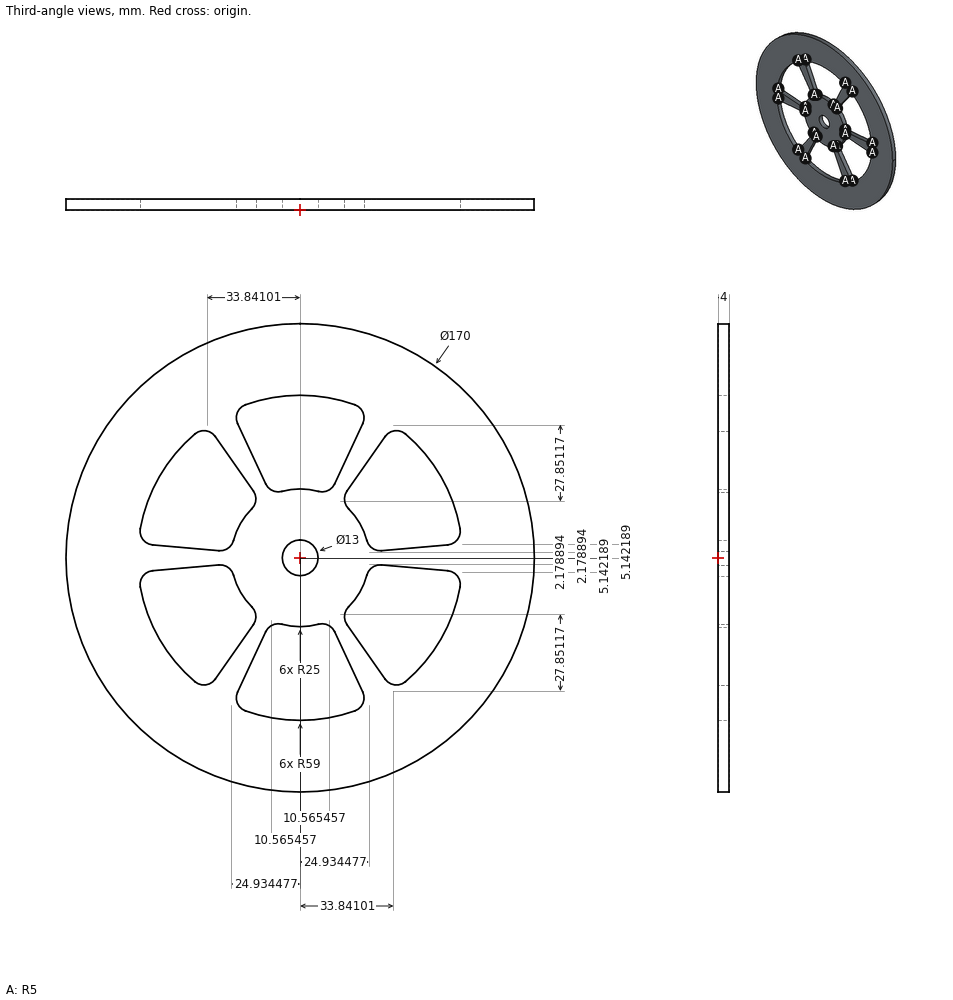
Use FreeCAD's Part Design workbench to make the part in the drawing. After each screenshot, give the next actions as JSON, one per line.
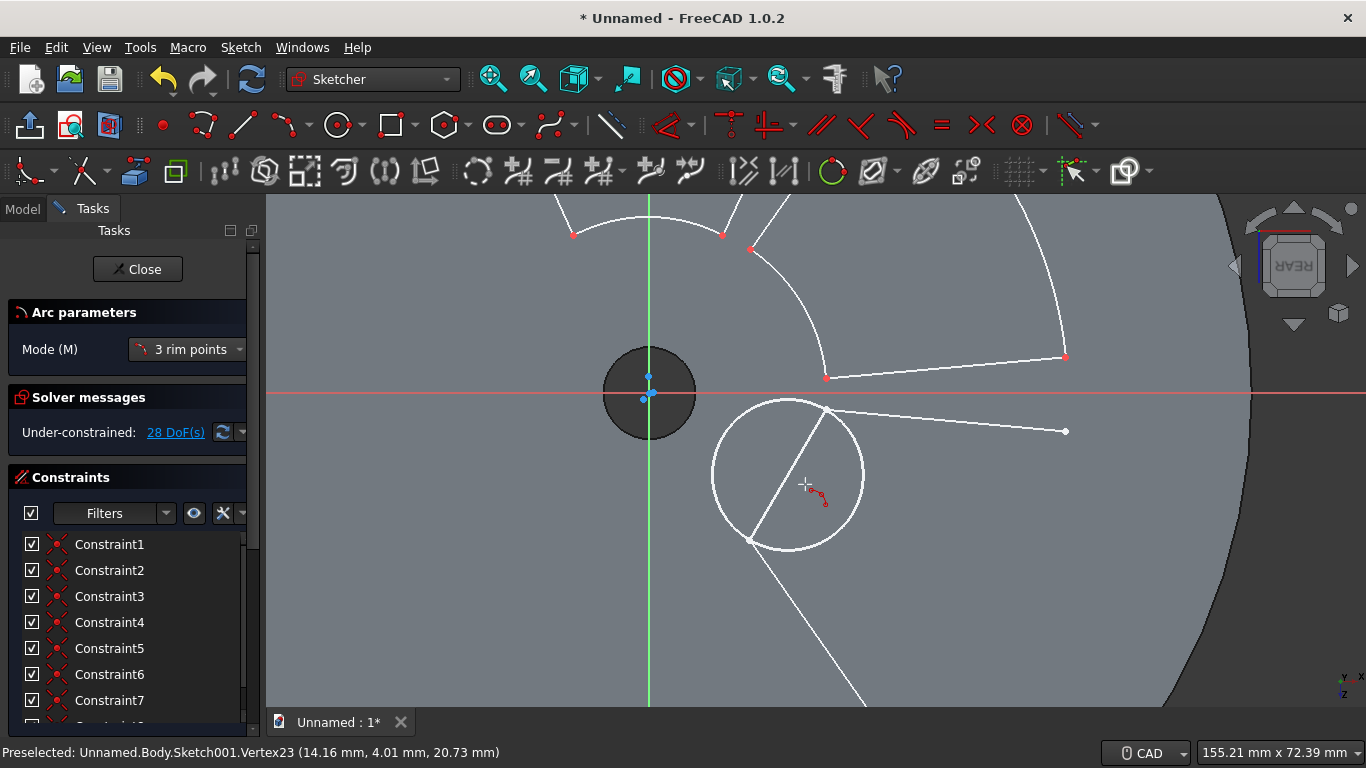
{"action": "left_click", "coordinate": [803, 482]}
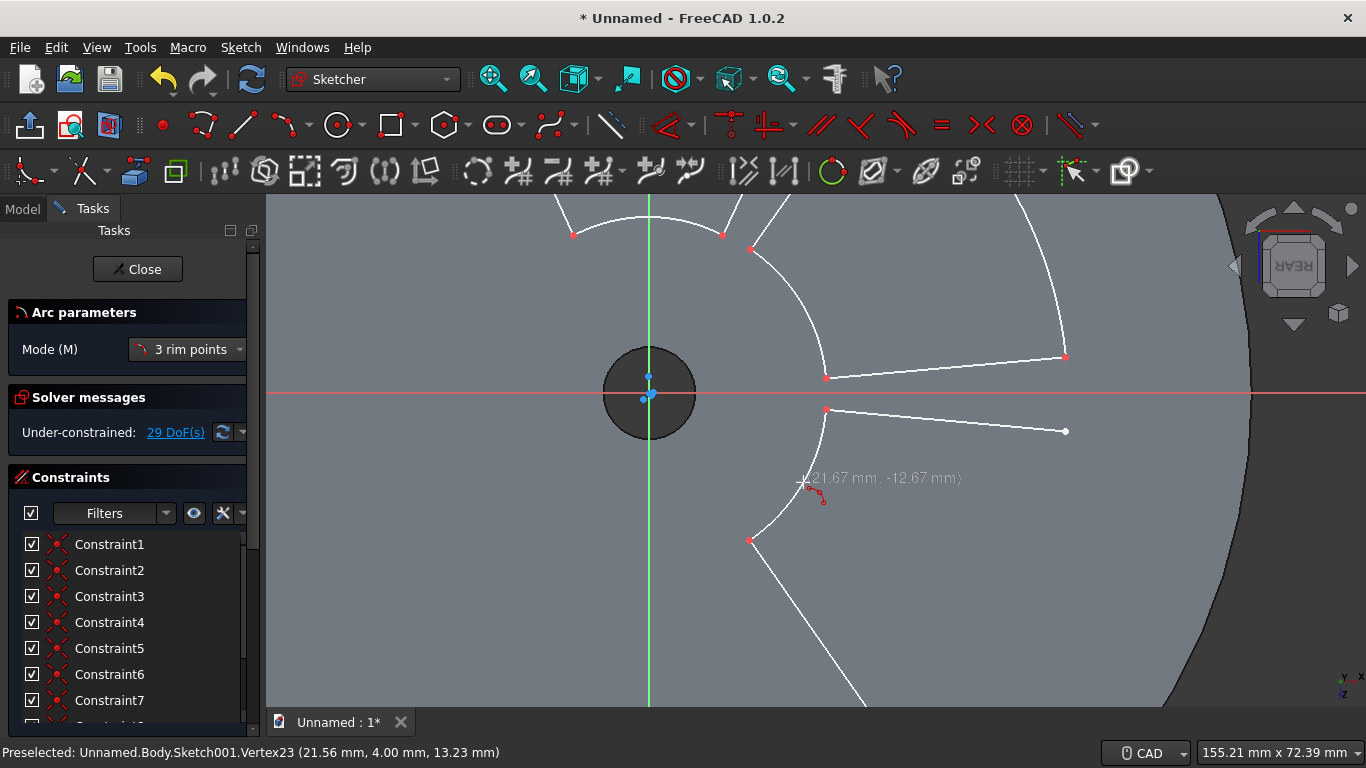
{"action": "scroll", "coordinate": [805, 484], "scroll_direction": "down", "scroll_amount": 5}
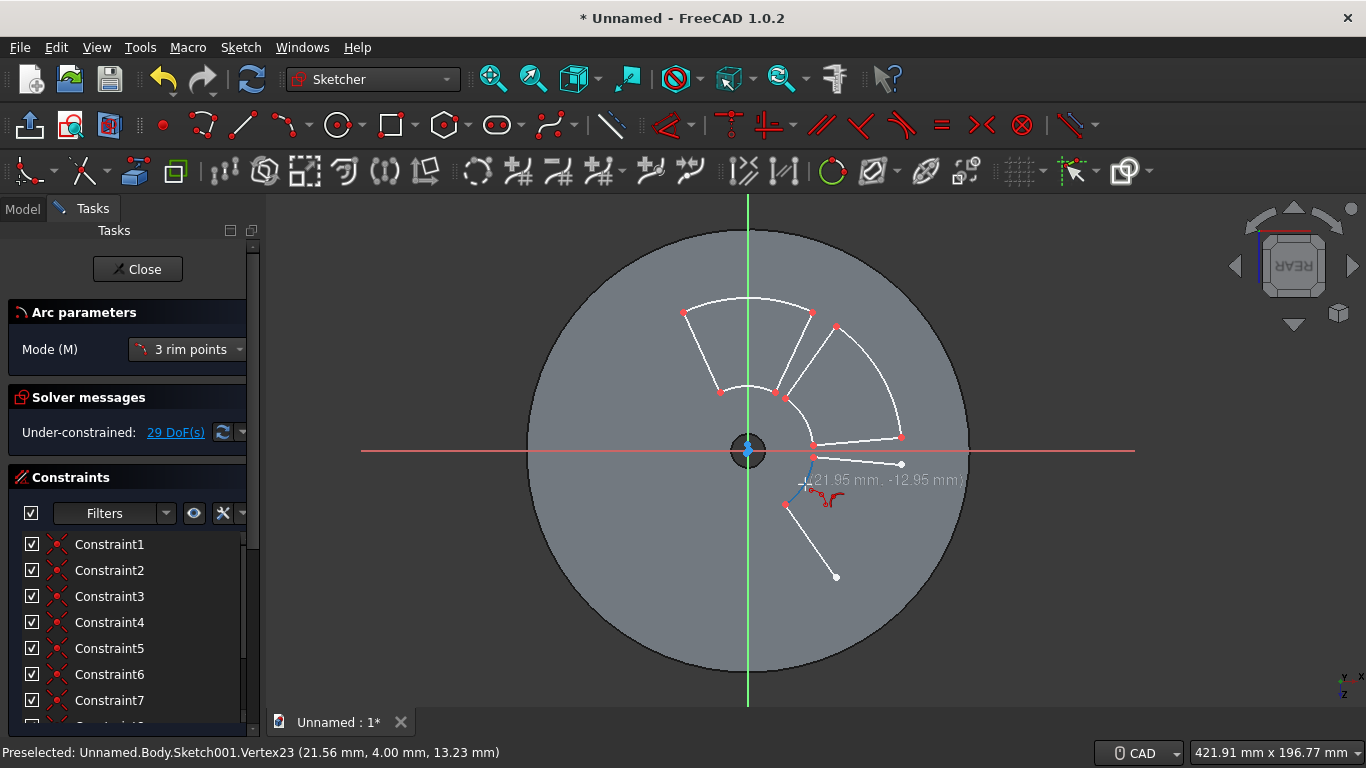
{"action": "left_click", "coordinate": [836, 578]}
{"action": "left_click", "coordinate": [901, 465]}
{"action": "left_click", "coordinate": [881, 528]}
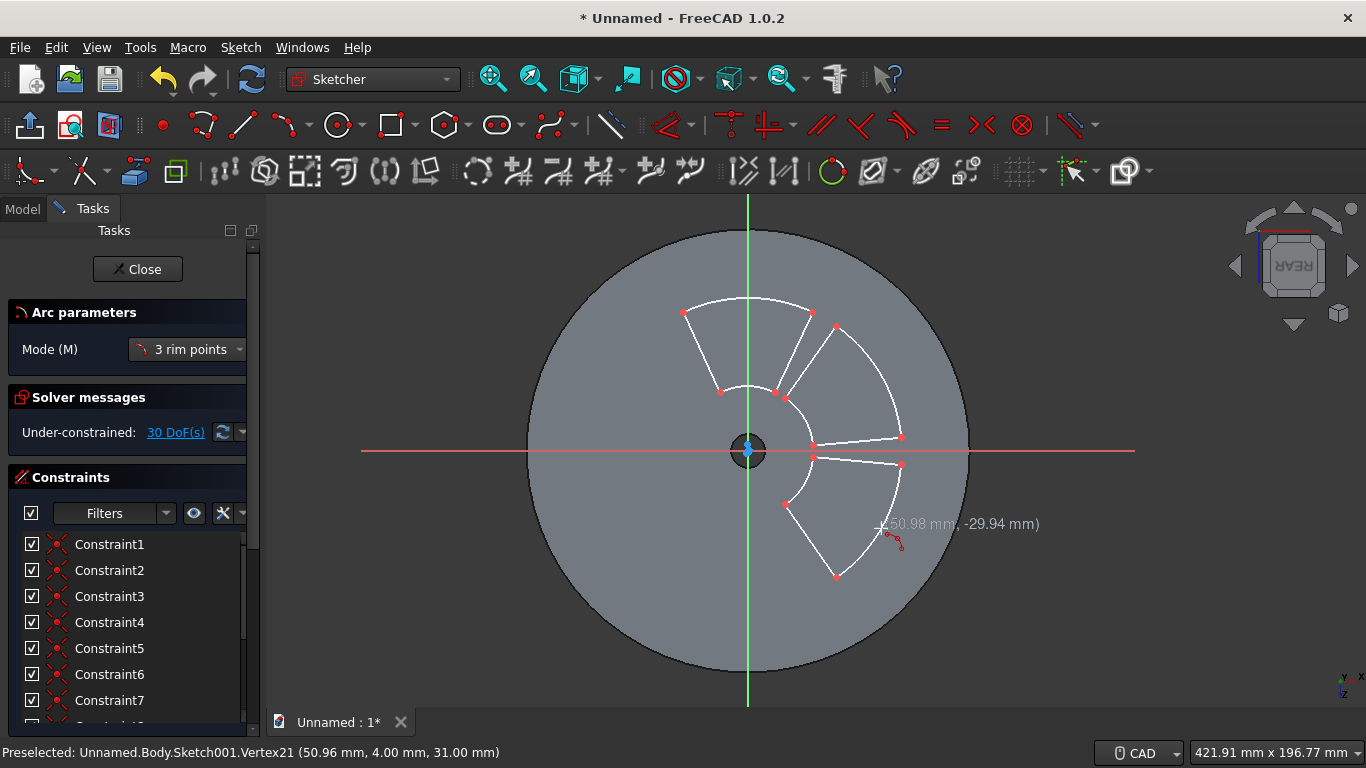
{"action": "left_click", "coordinate": [244, 126]}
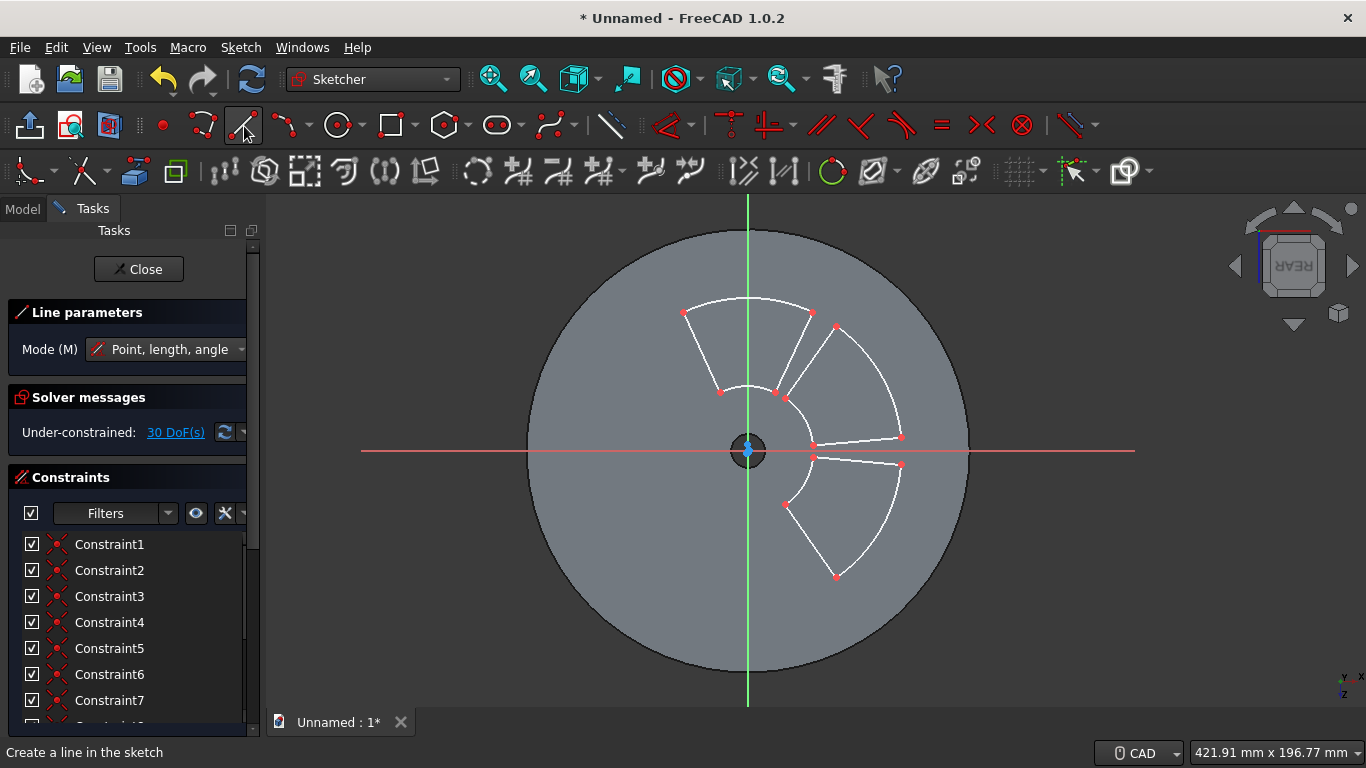
{"action": "left_click", "coordinate": [813, 590]}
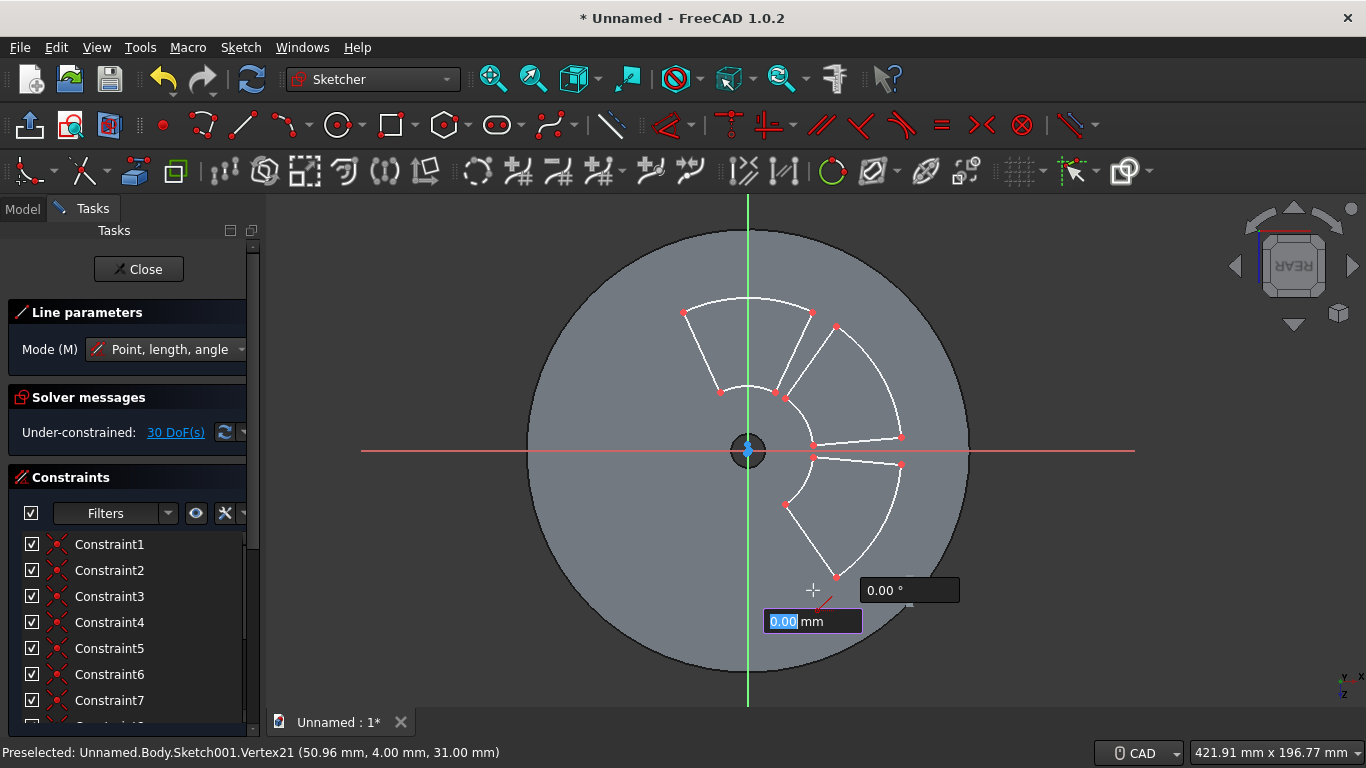
{"action": "scroll", "coordinate": [776, 510], "scroll_direction": "up", "scroll_amount": 2}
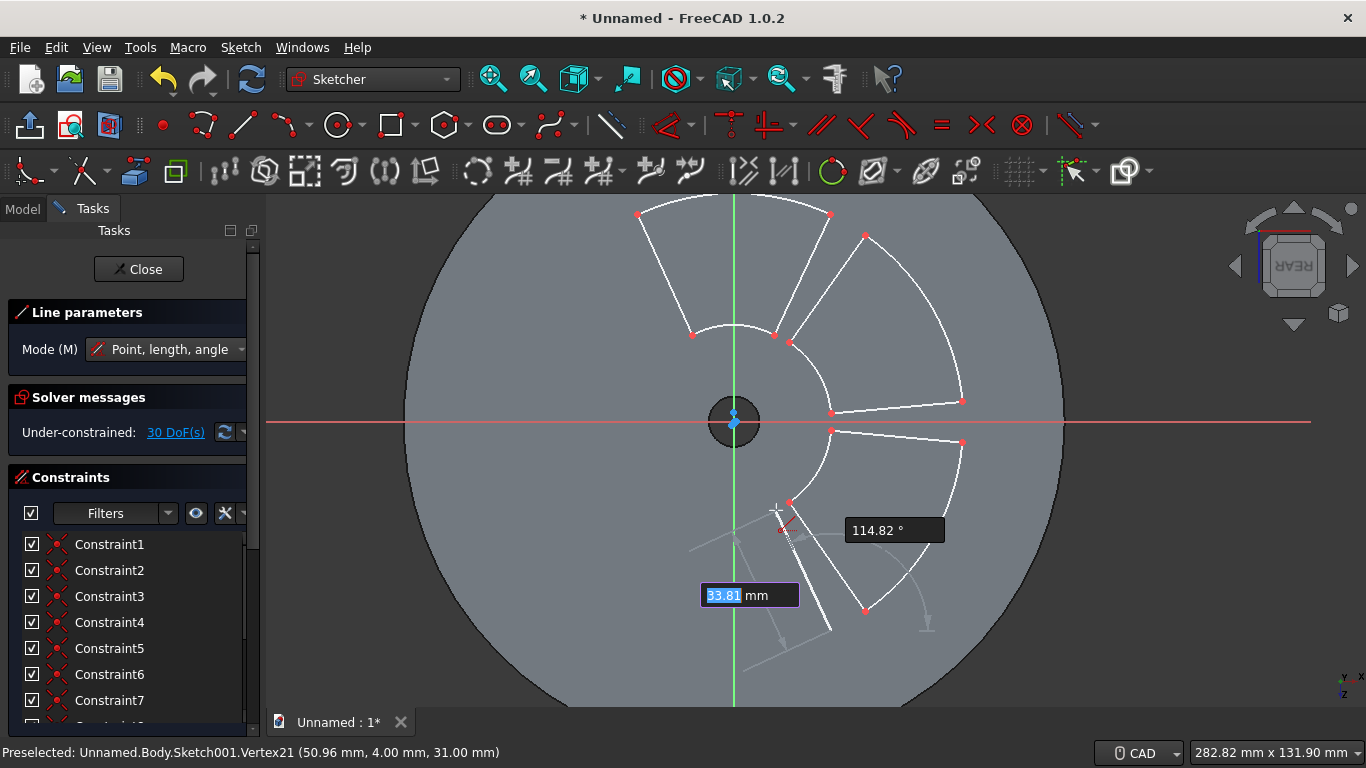
{"action": "left_click", "coordinate": [775, 510]}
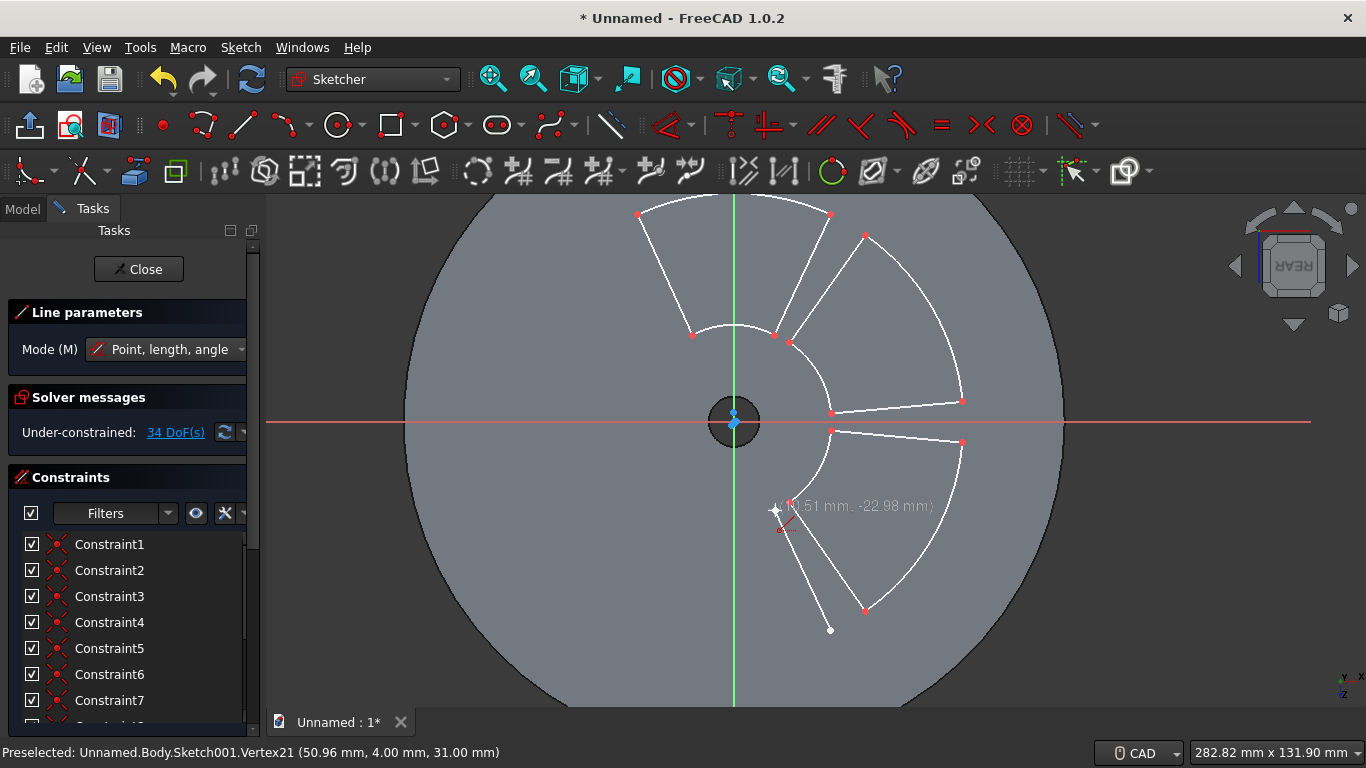
{"action": "left_click", "coordinate": [693, 510]}
{"action": "left_click", "coordinate": [637, 630]}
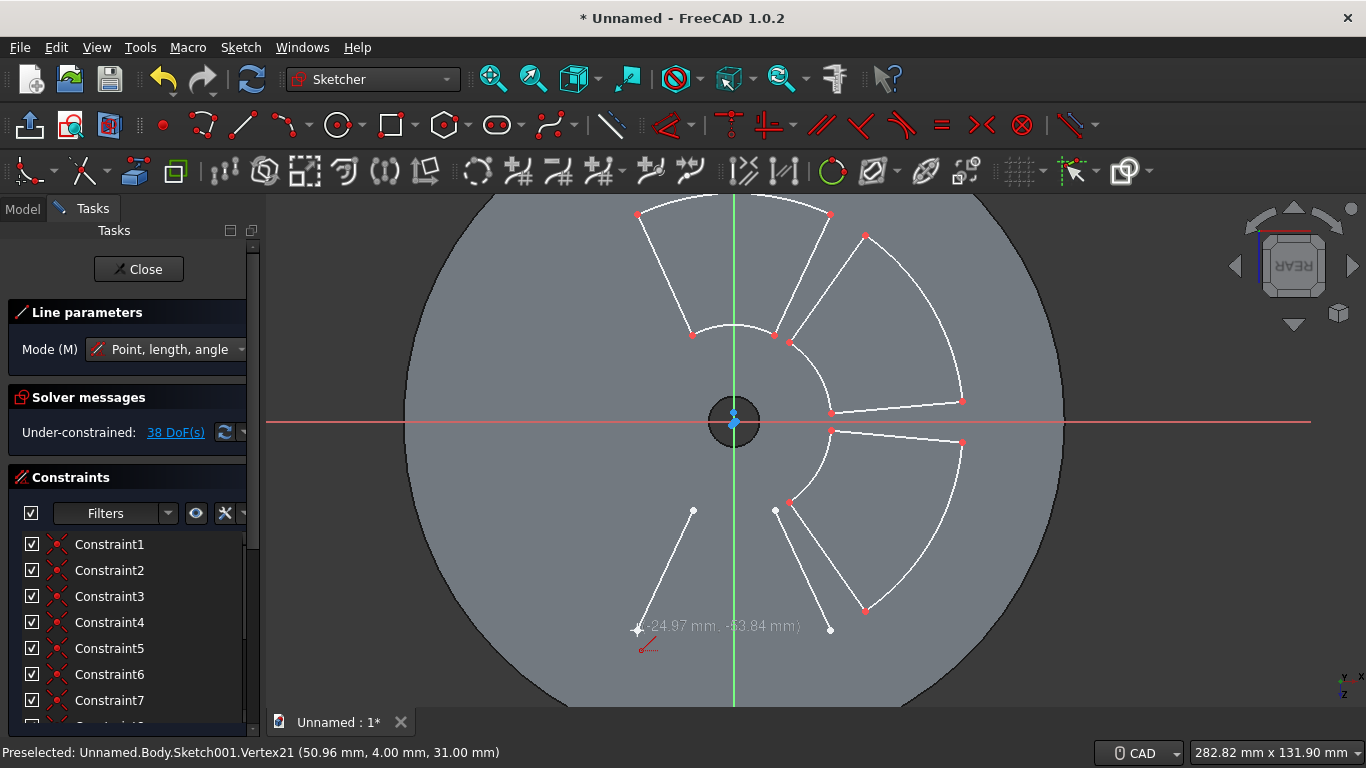
{"action": "left_click", "coordinate": [284, 126]}